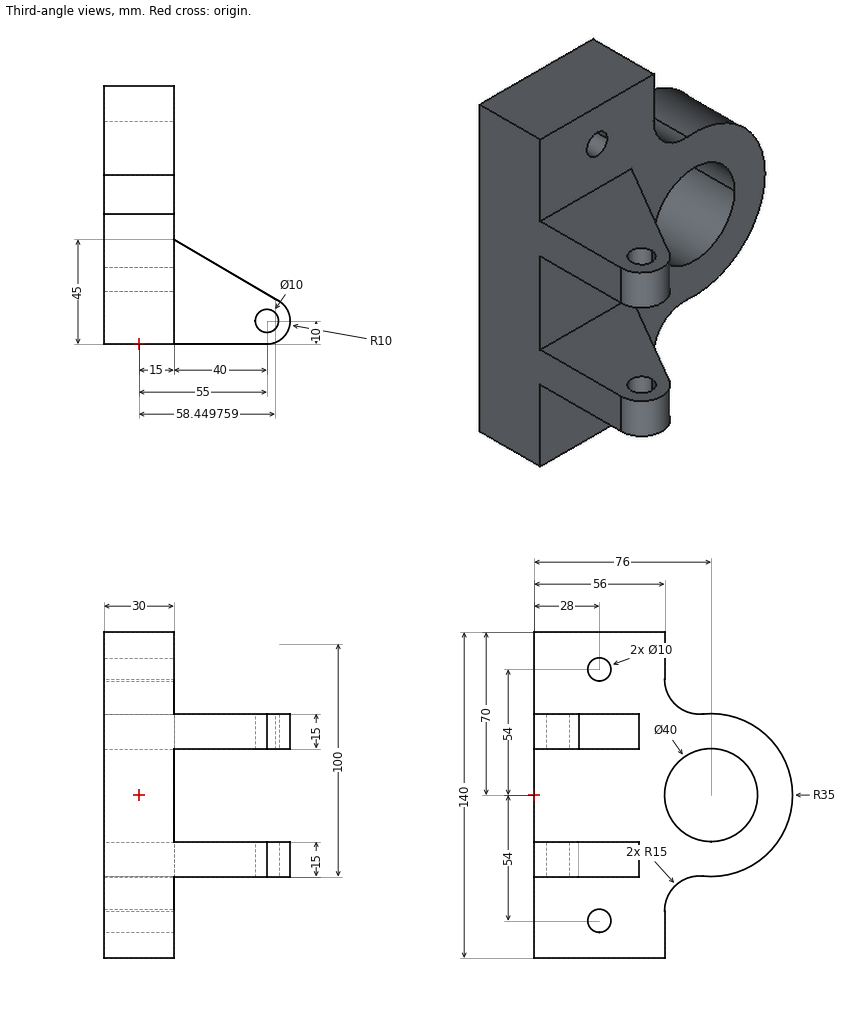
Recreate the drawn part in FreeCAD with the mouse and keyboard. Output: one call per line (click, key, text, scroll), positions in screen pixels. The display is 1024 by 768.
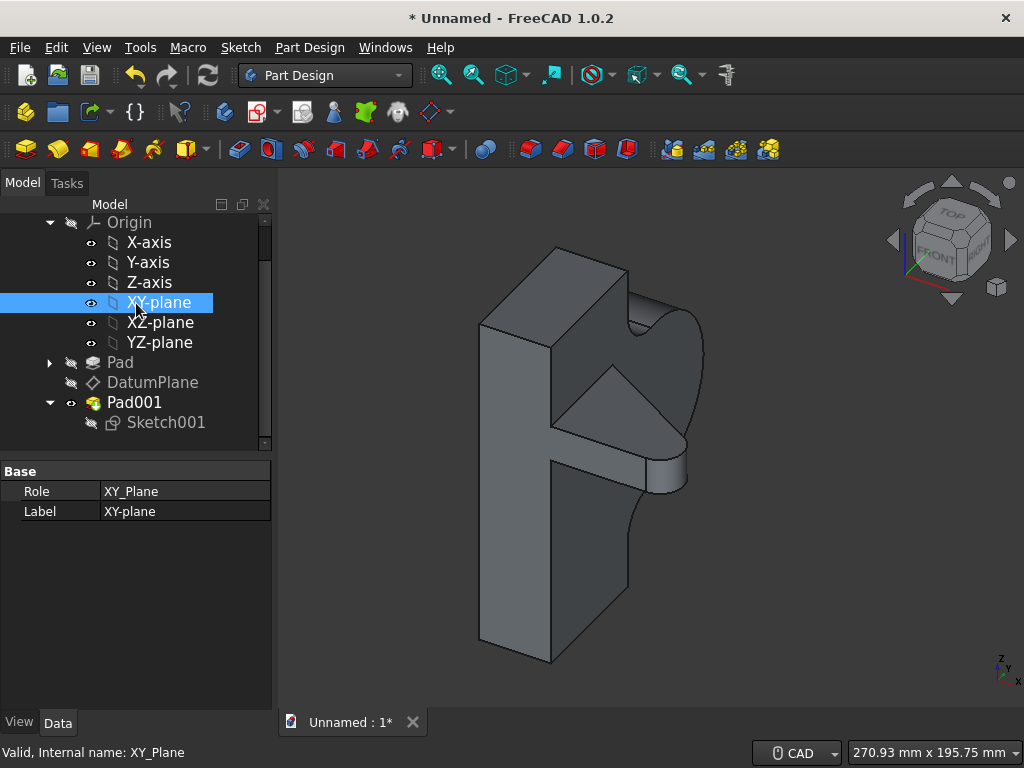
click(430, 112)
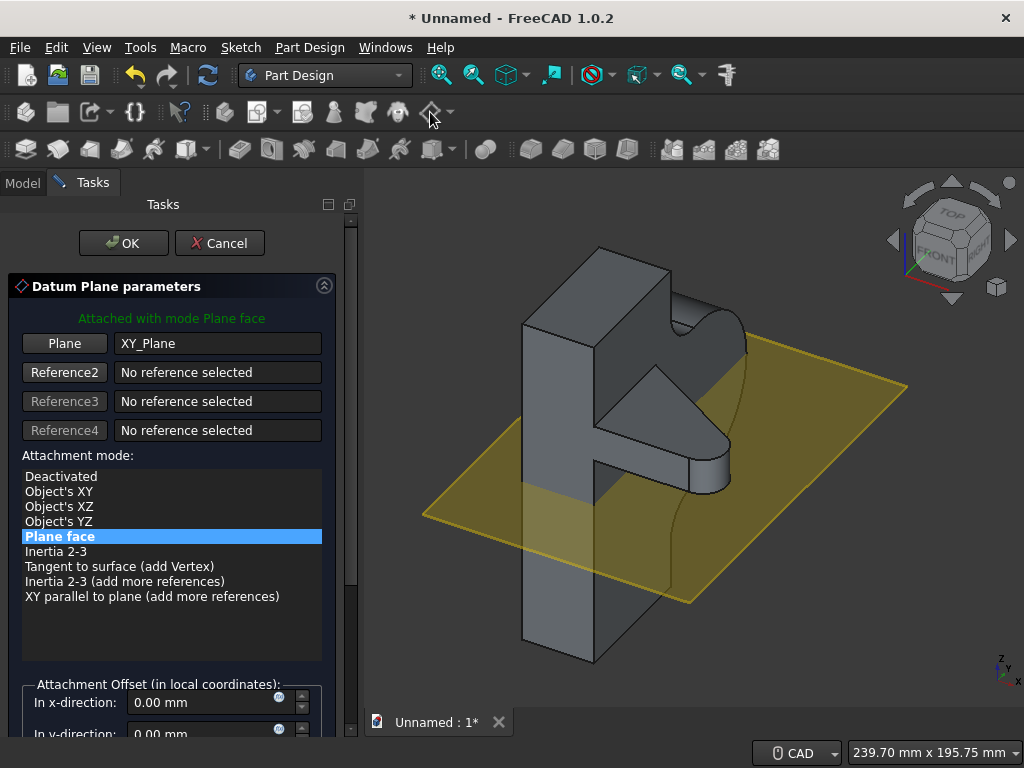
scroll(351, 475, down, 2)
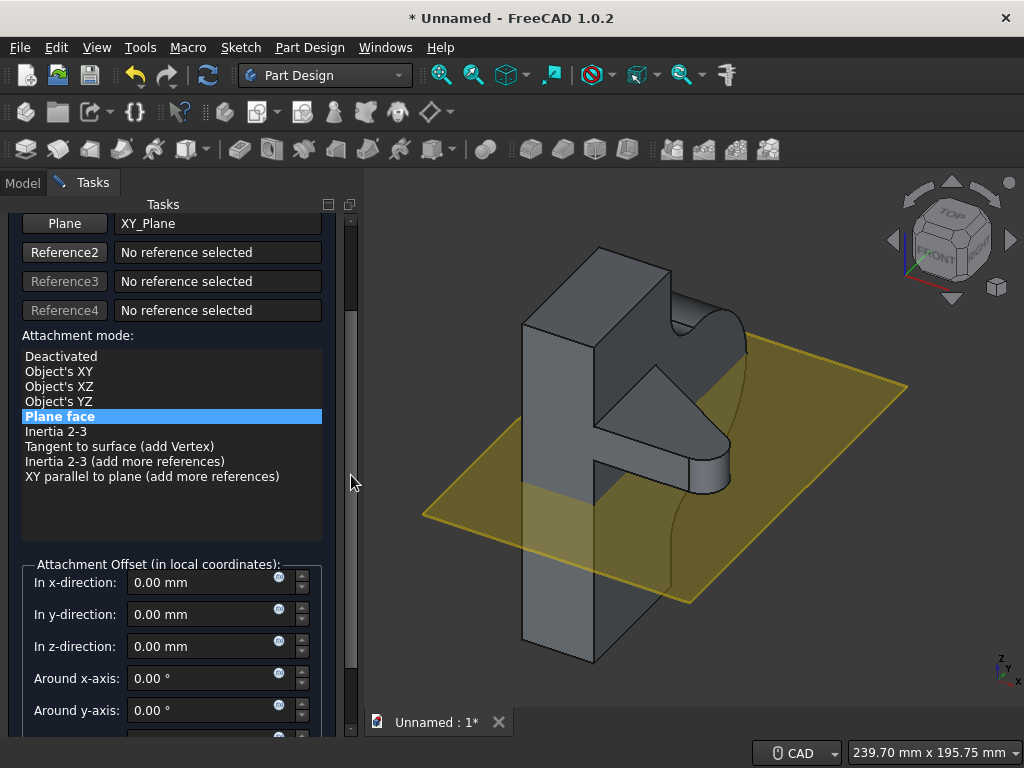
triple_click(210, 646)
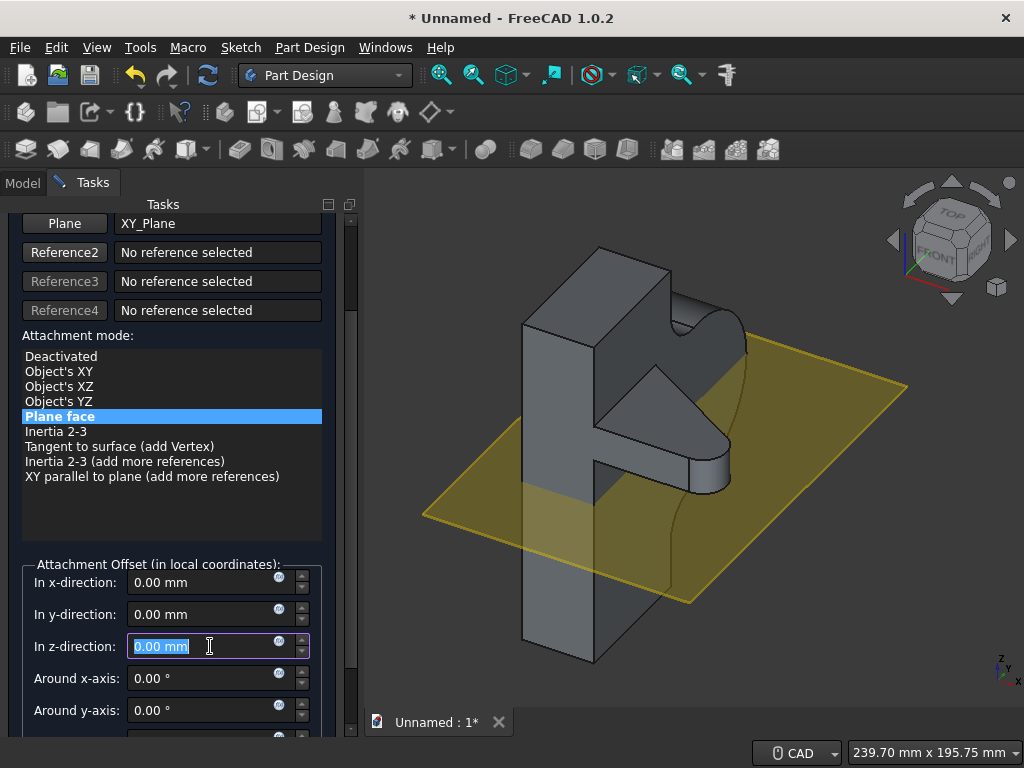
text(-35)
key(Tab)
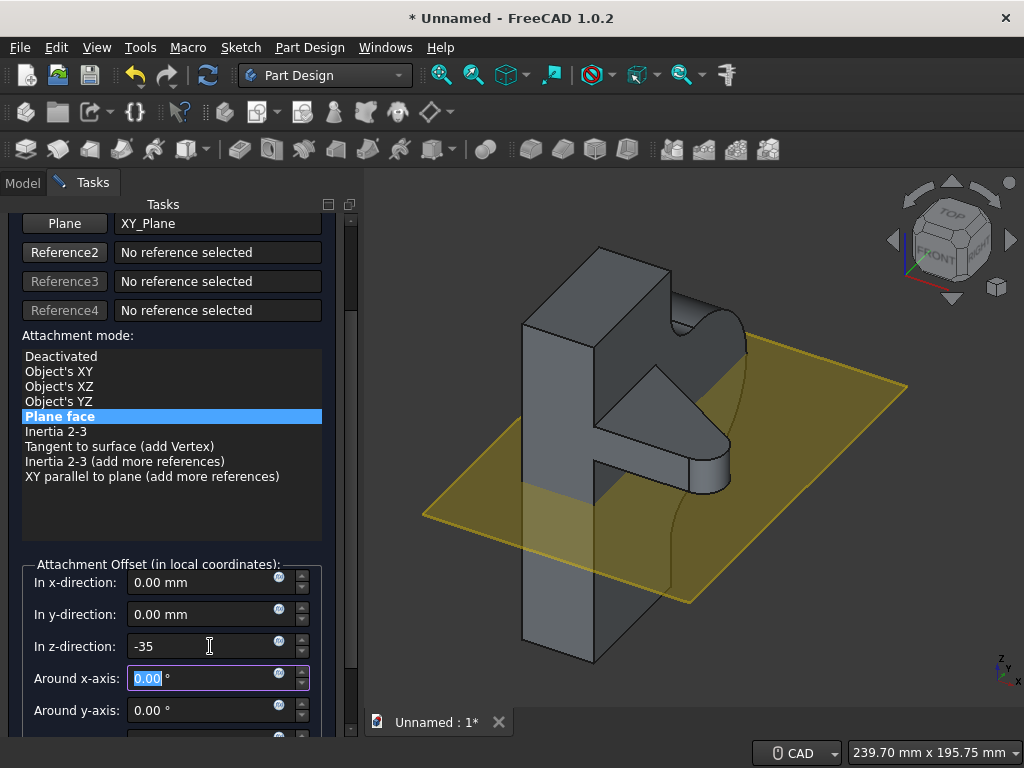
scroll(351, 475, up, 3)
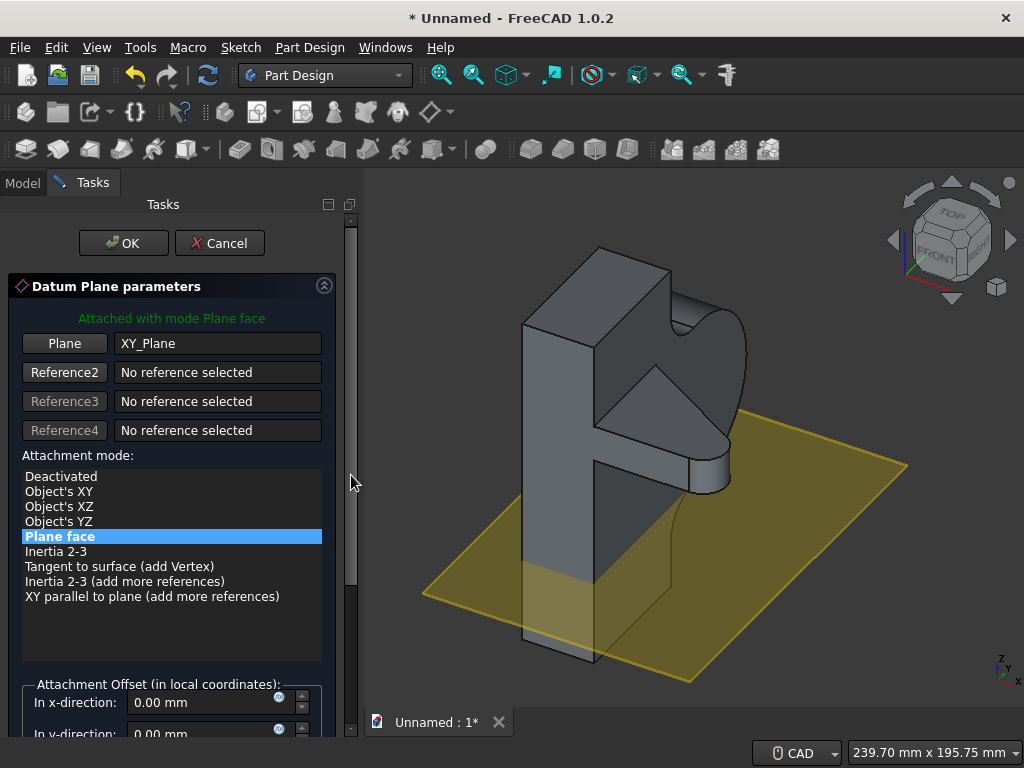
click(124, 243)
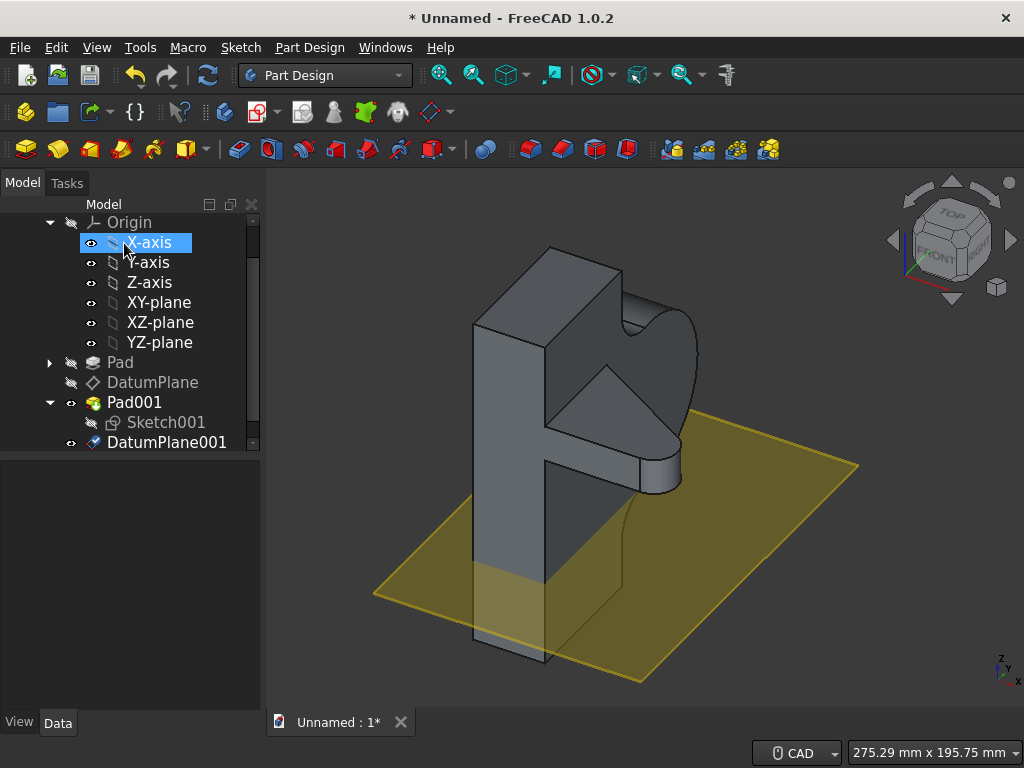
click(116, 443)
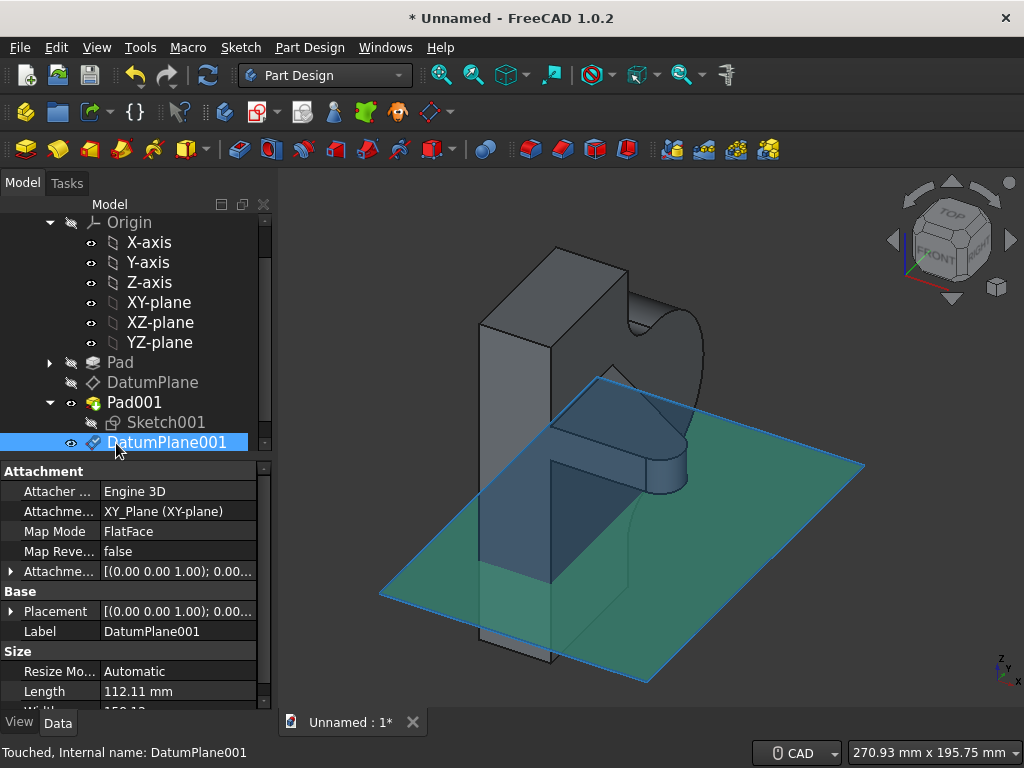
click(258, 112)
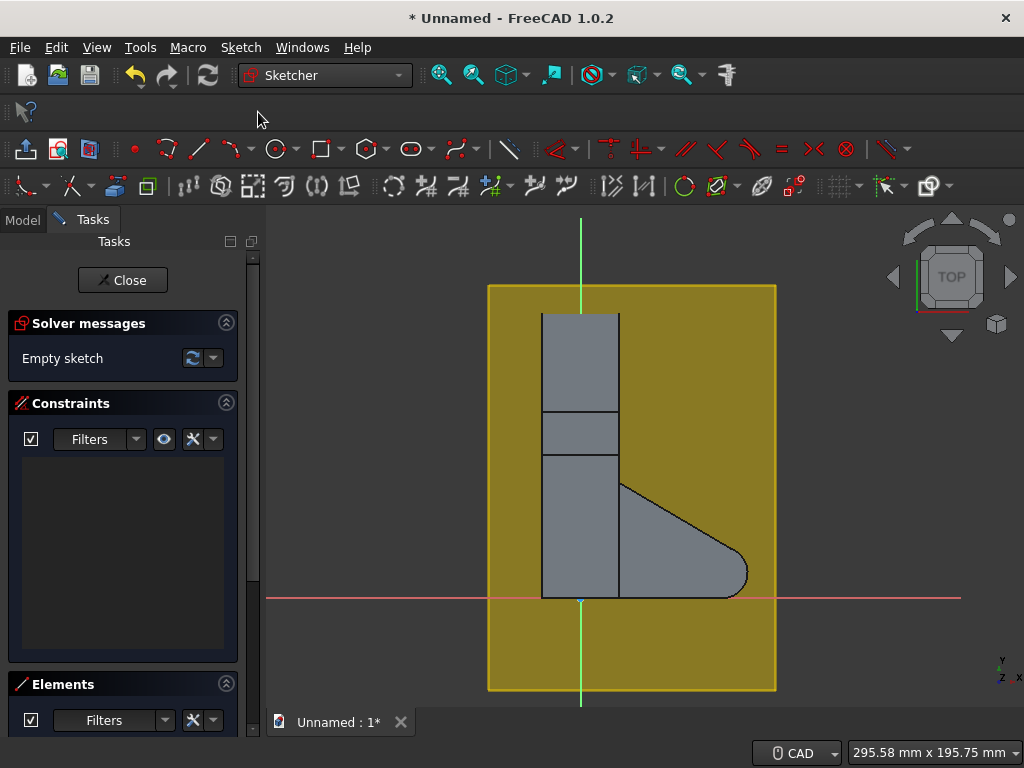
key(q)
key(s)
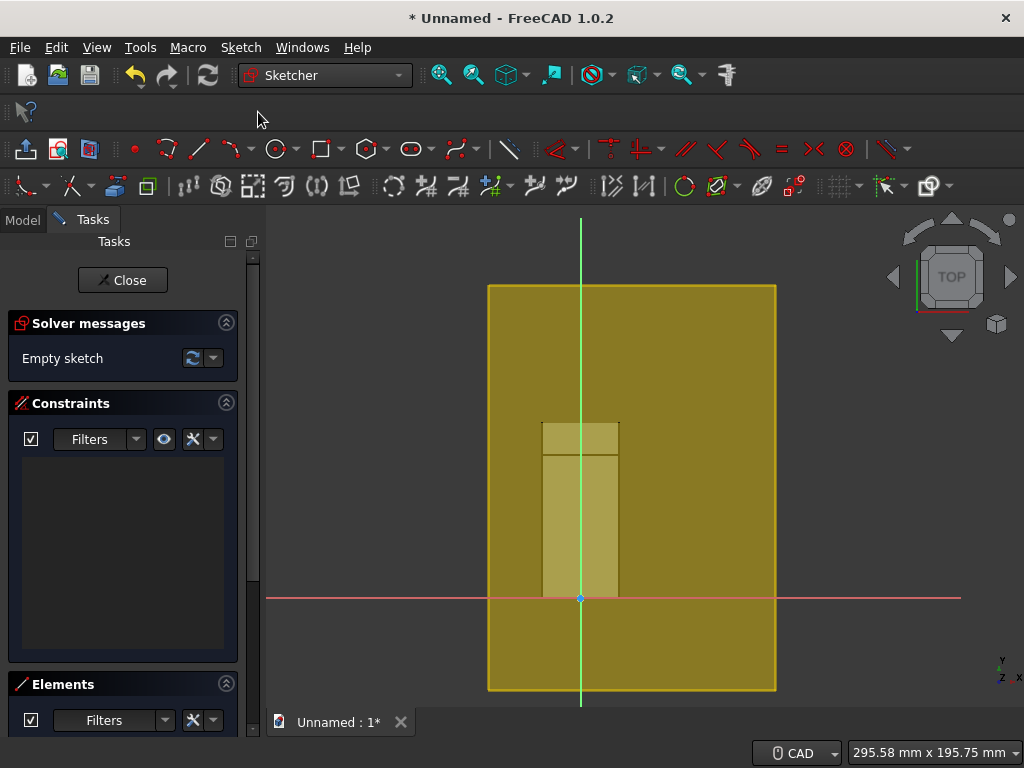
scroll(735, 610, up, 4)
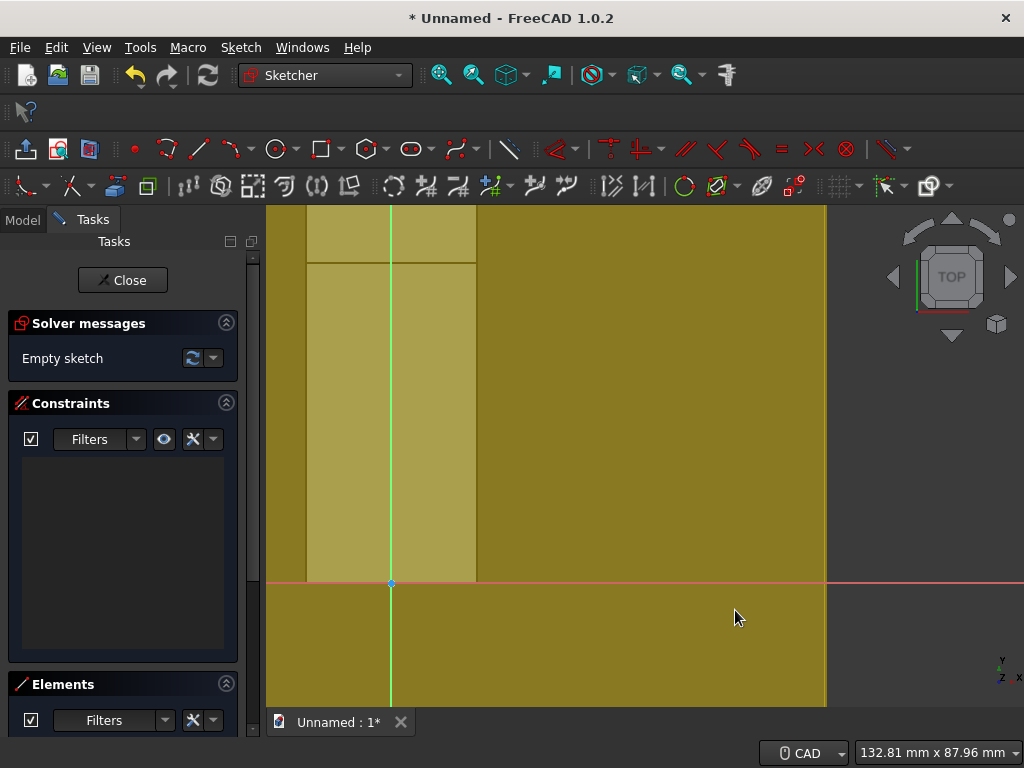
key(g)
key(m)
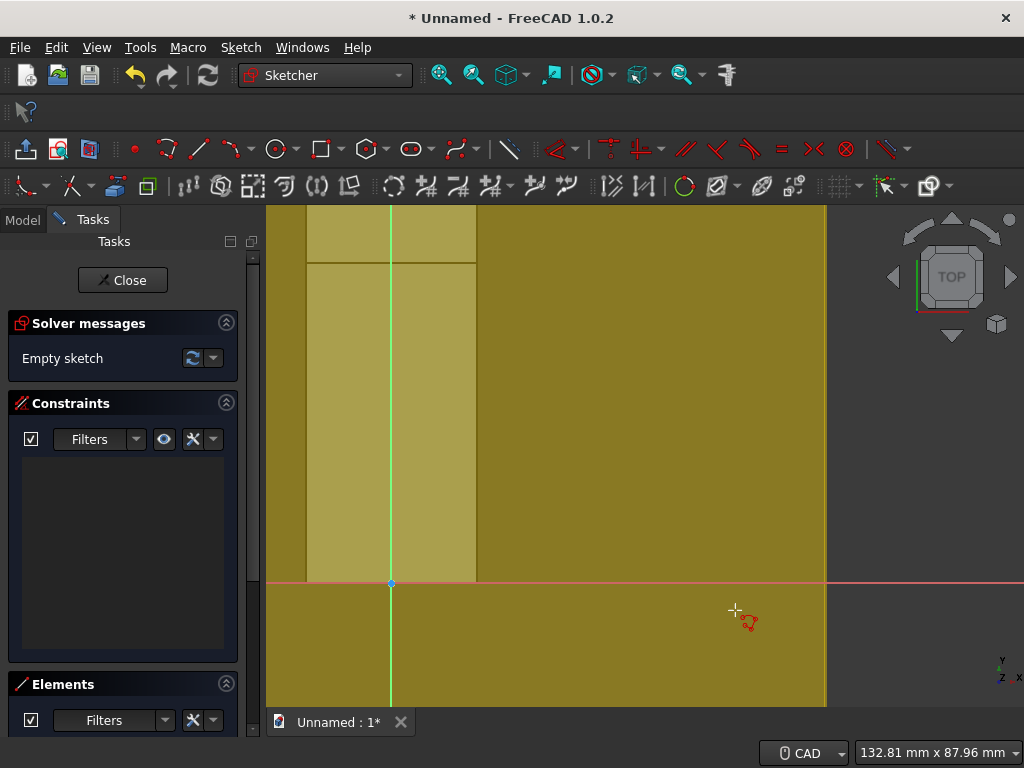
click(734, 477)
click(477, 326)
click(477, 583)
click(705, 574)
right_click(705, 574)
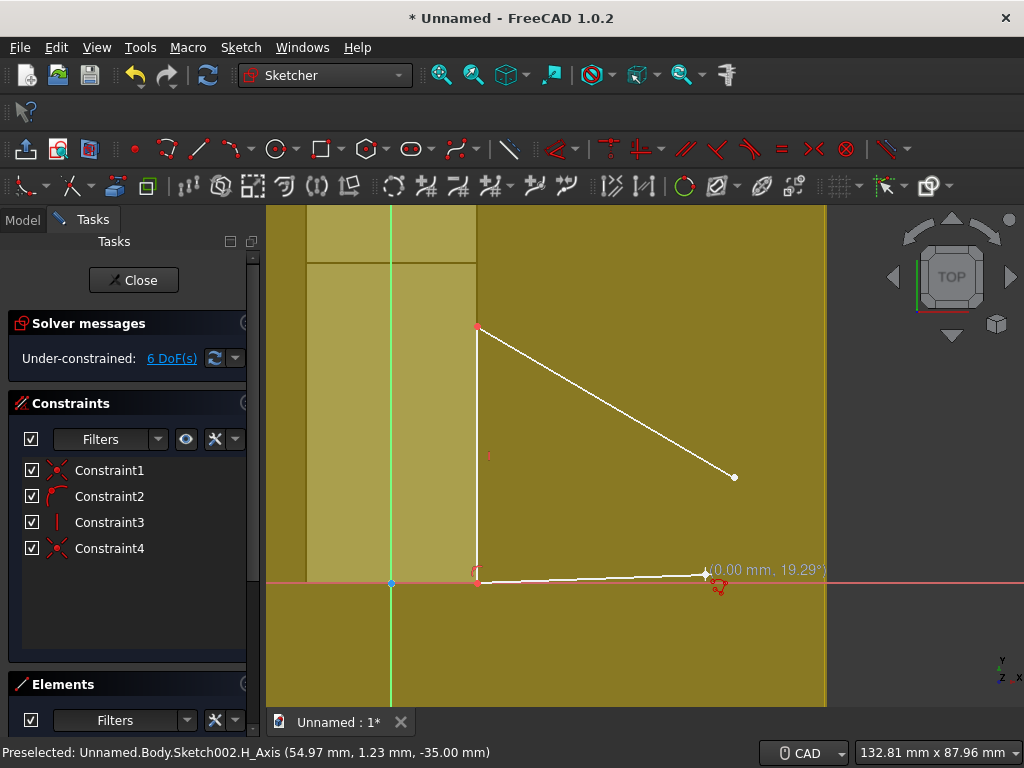
click(232, 150)